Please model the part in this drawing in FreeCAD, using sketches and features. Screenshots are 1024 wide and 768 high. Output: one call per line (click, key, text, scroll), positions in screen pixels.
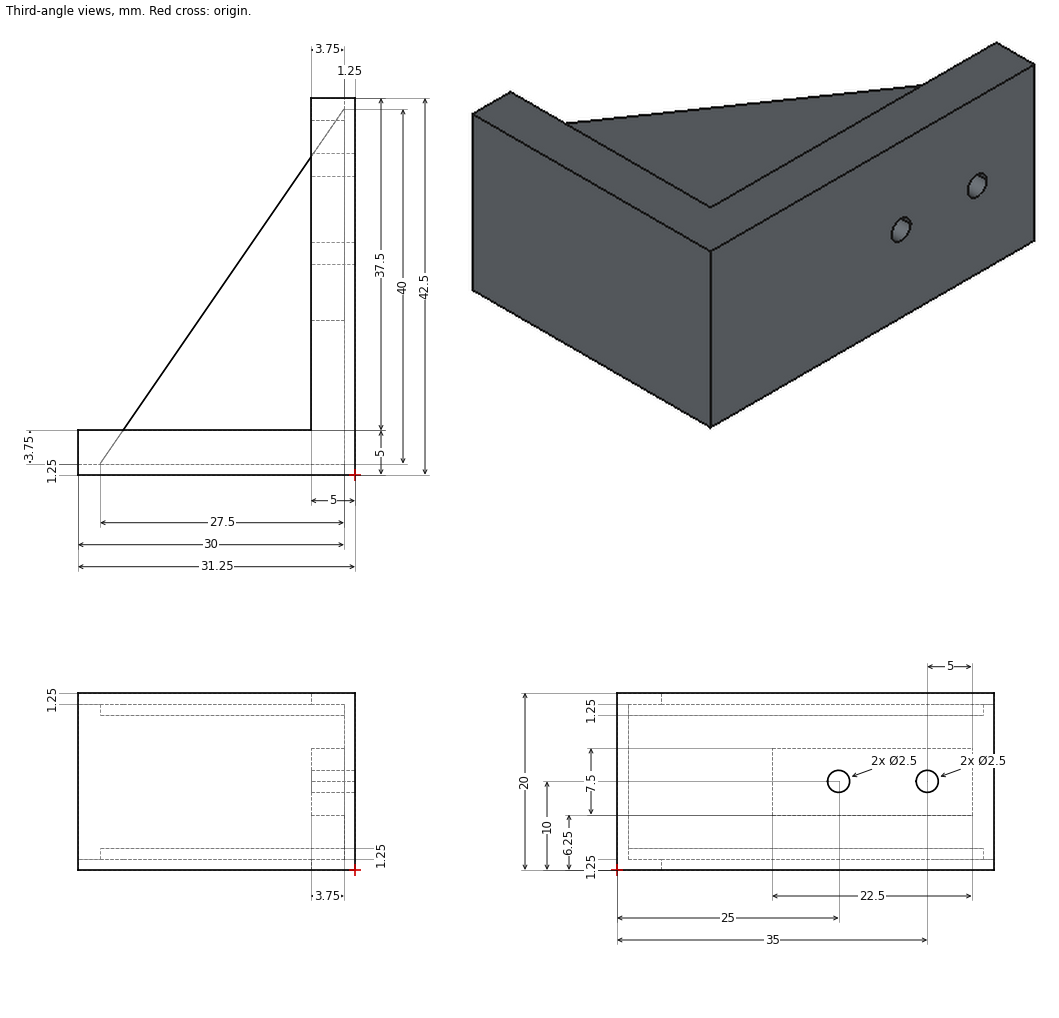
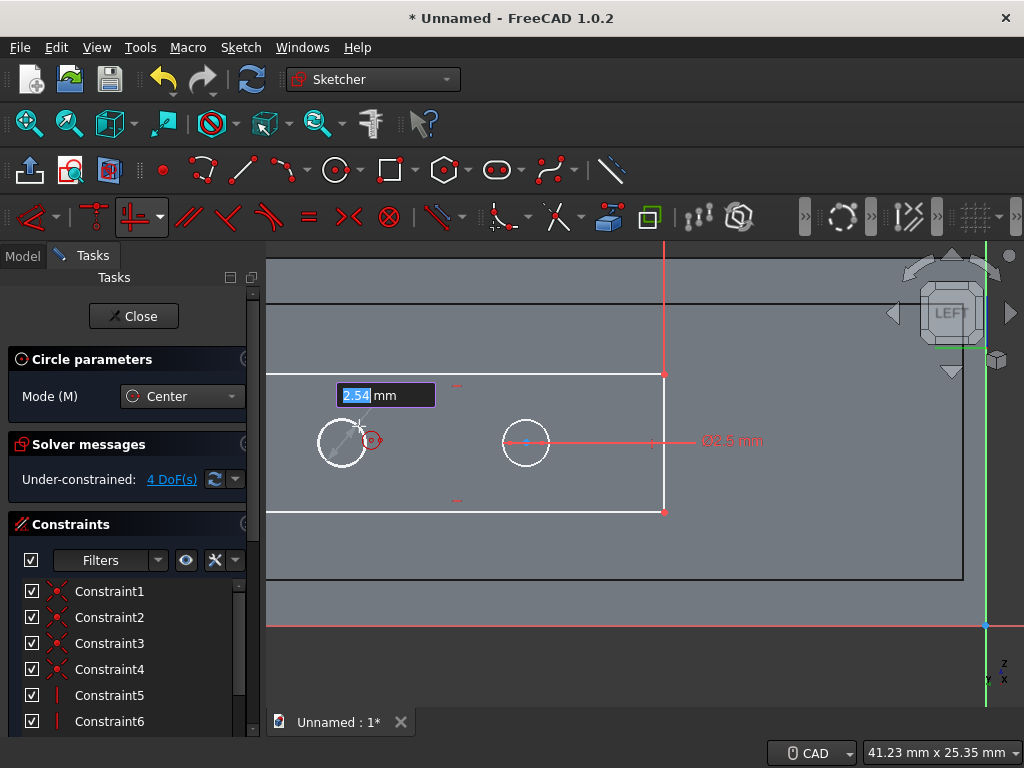
text(2.5)
key(Return)
key(Escape)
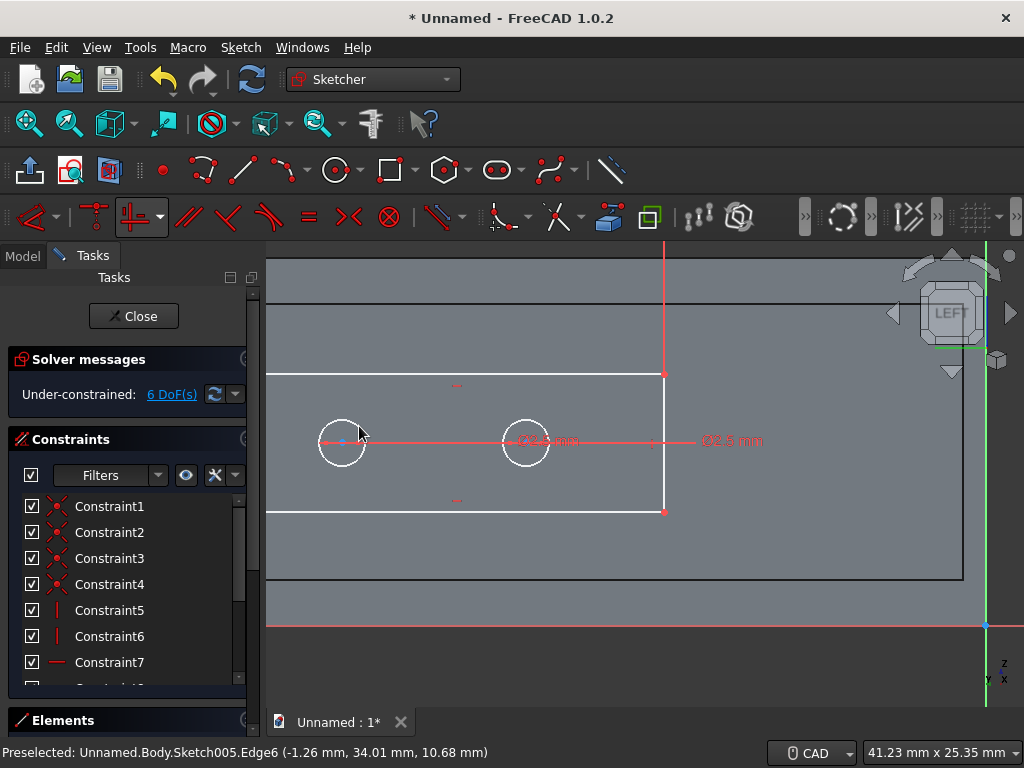
click(526, 443)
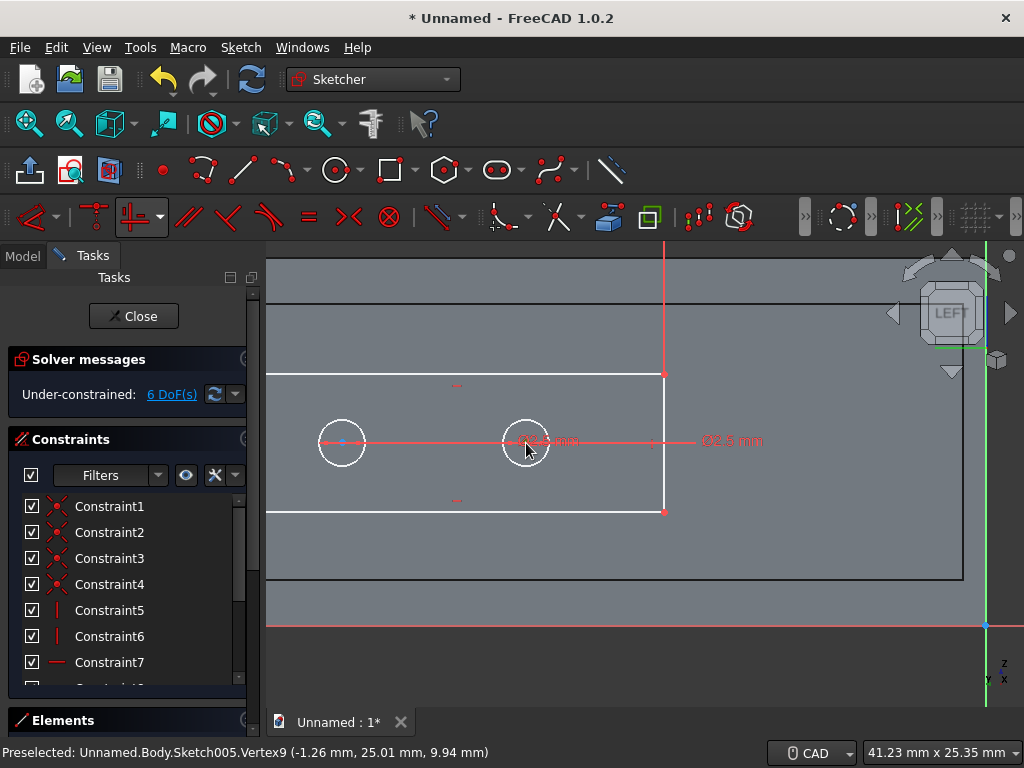
click(342, 443)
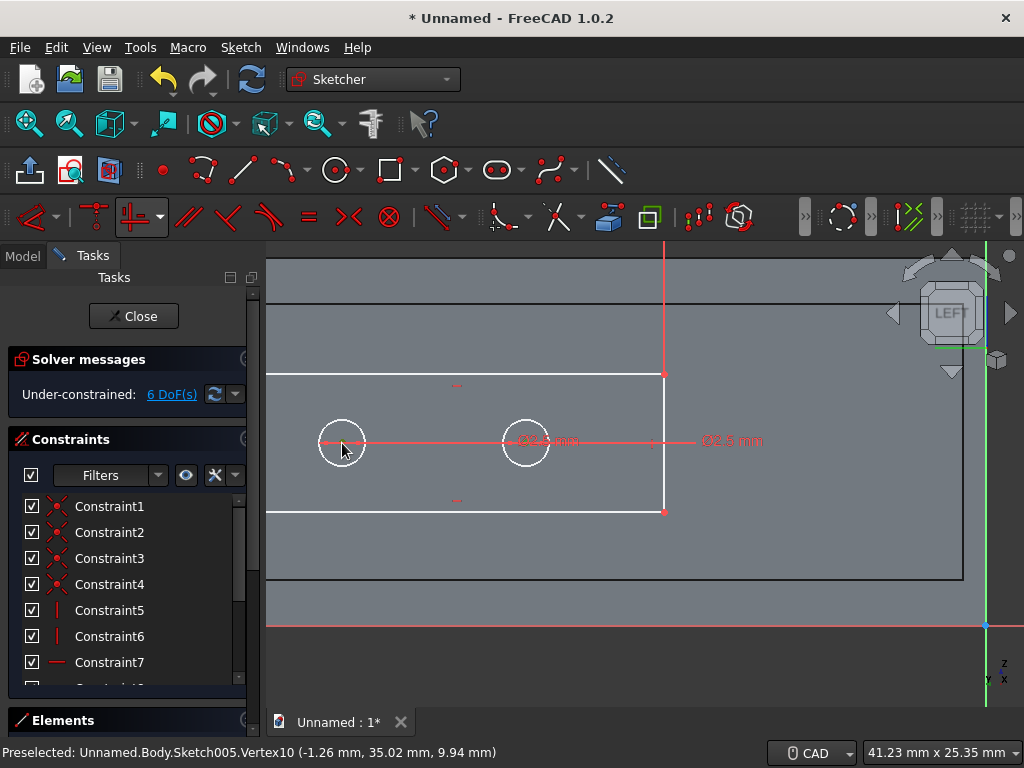
key(h)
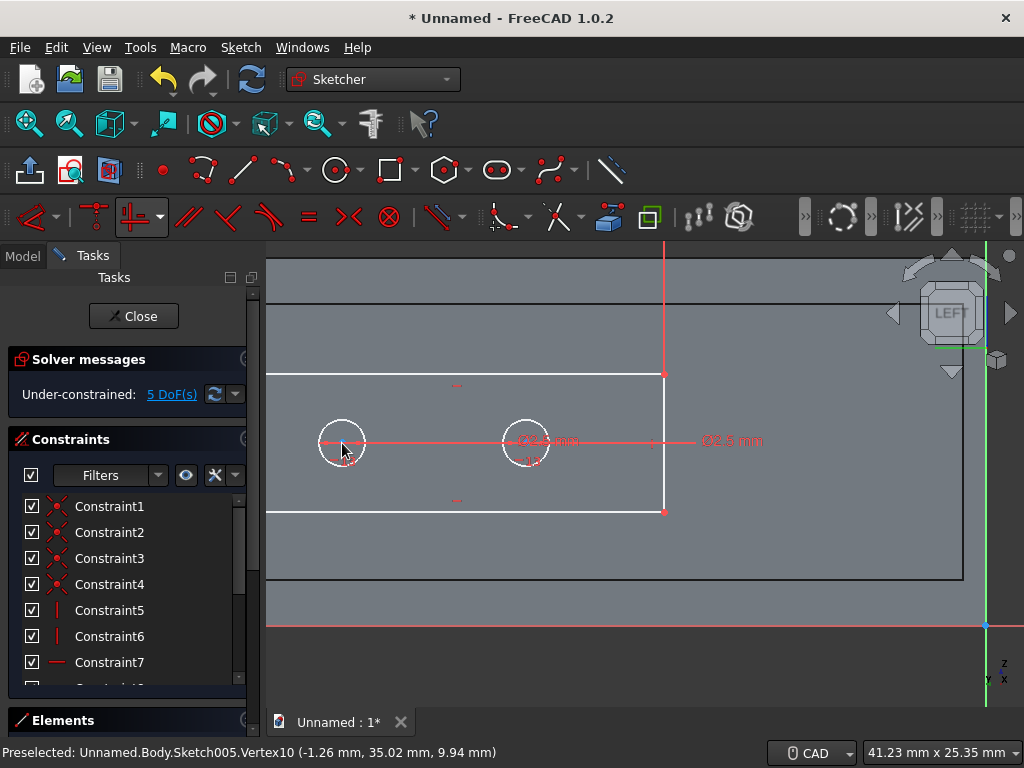
click(32, 218)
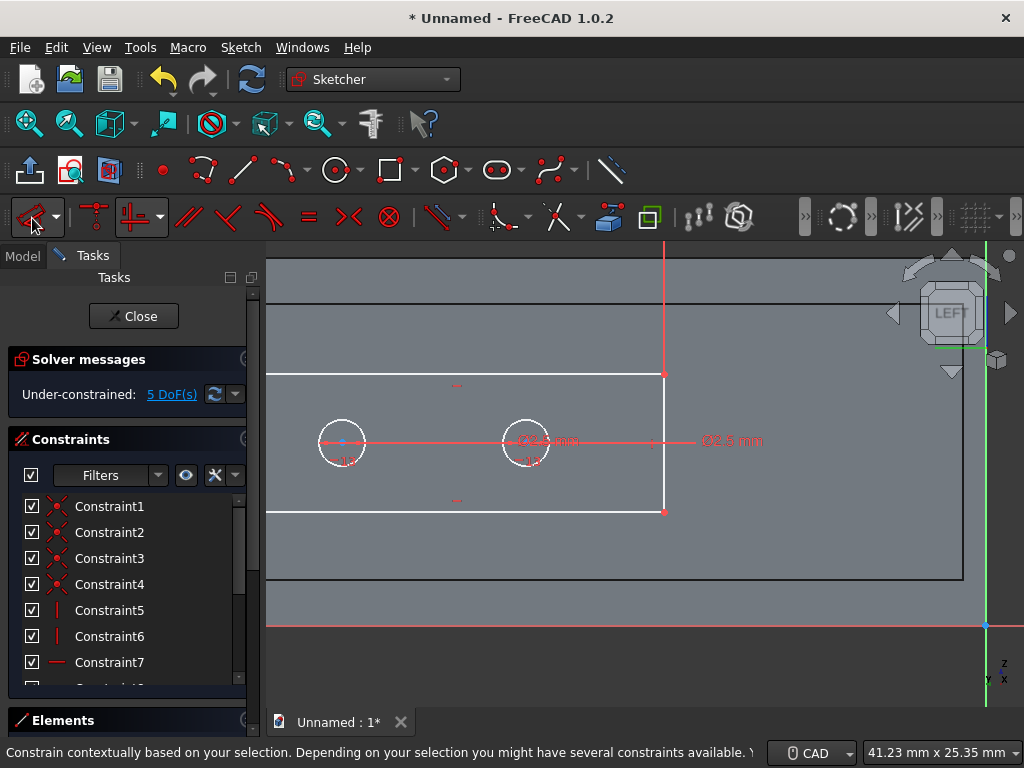
click(526, 443)
click(692, 660)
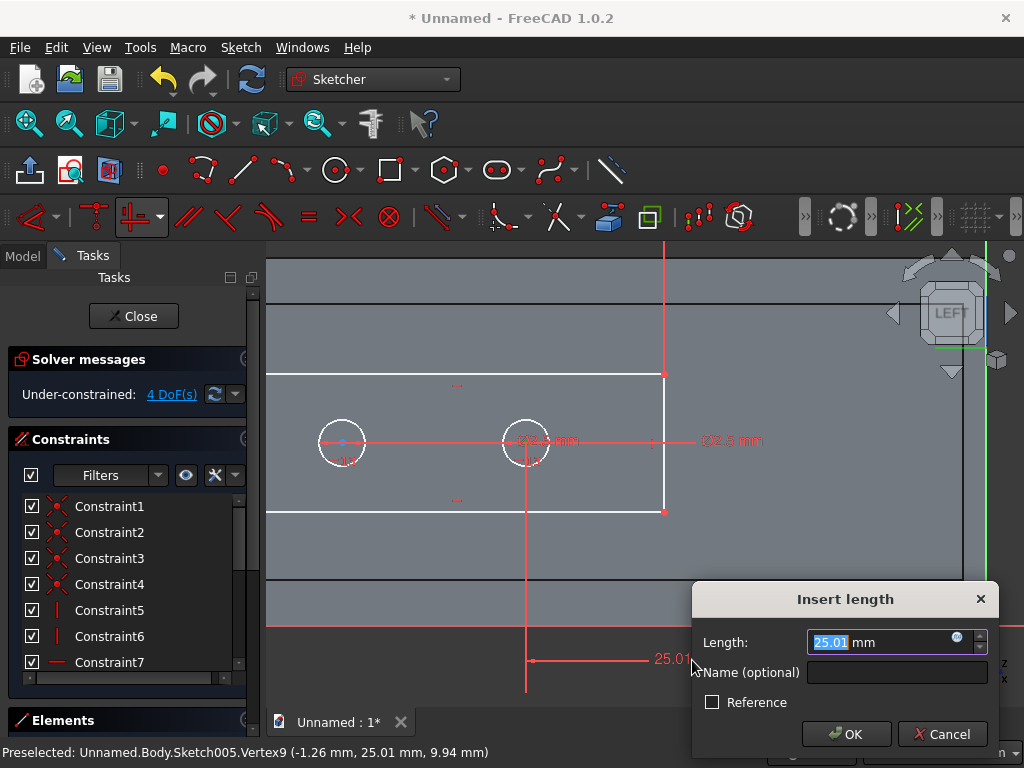
text(25)
key(Return)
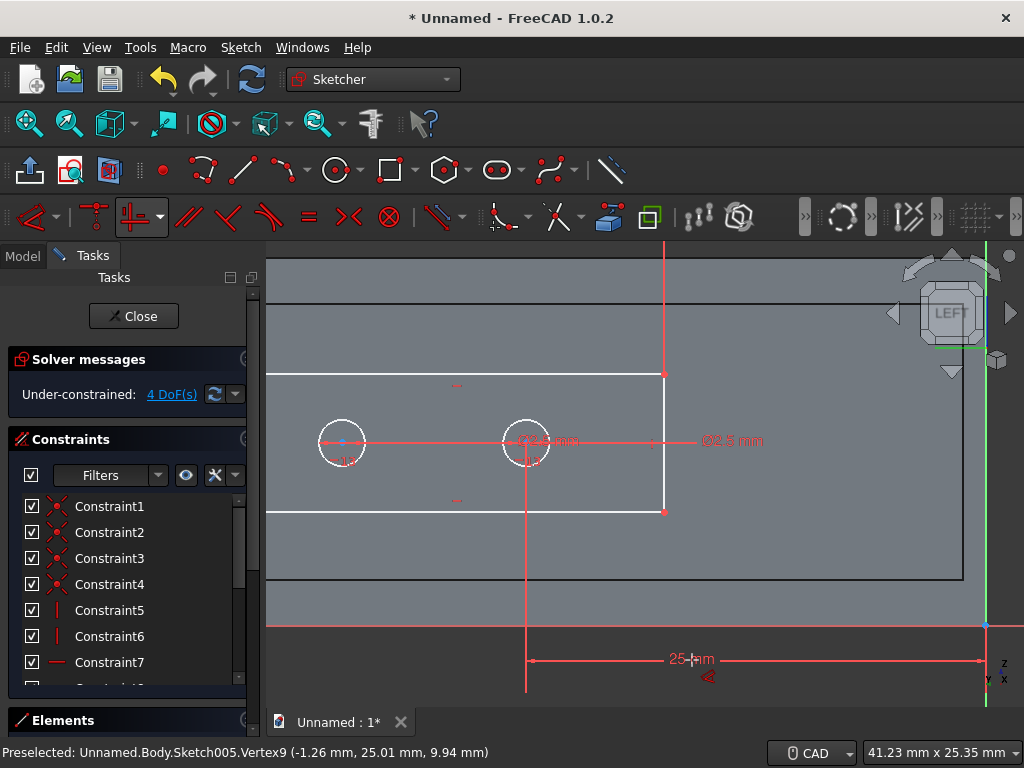
click(526, 443)
click(492, 534)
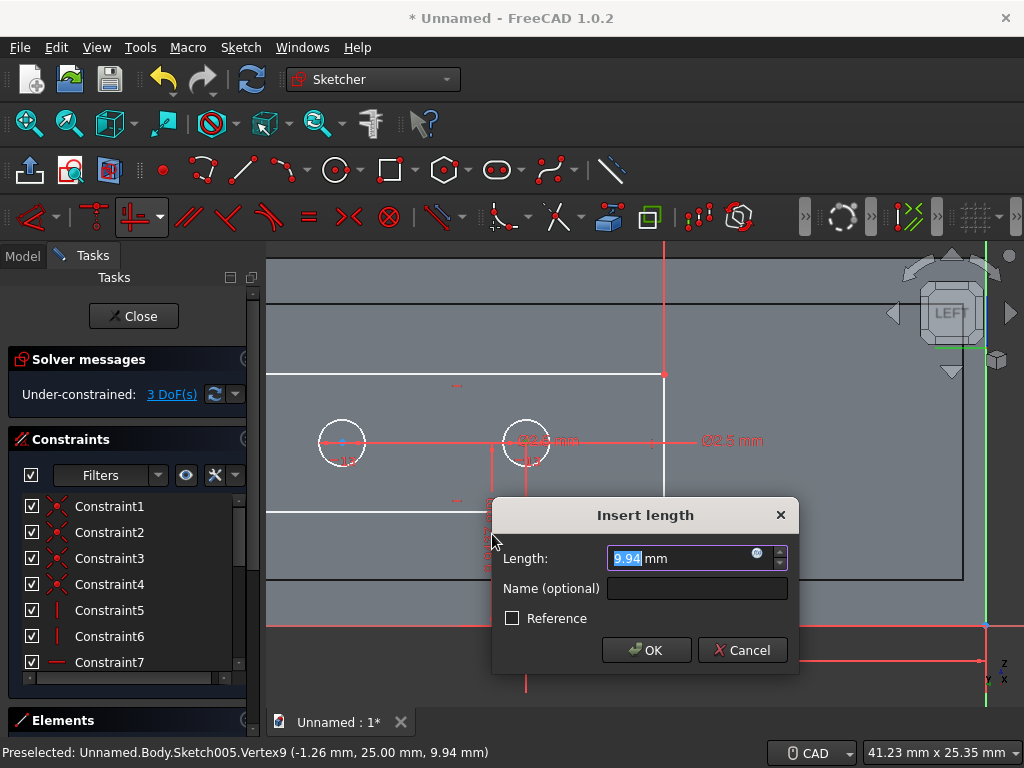
text(10)
key(Return)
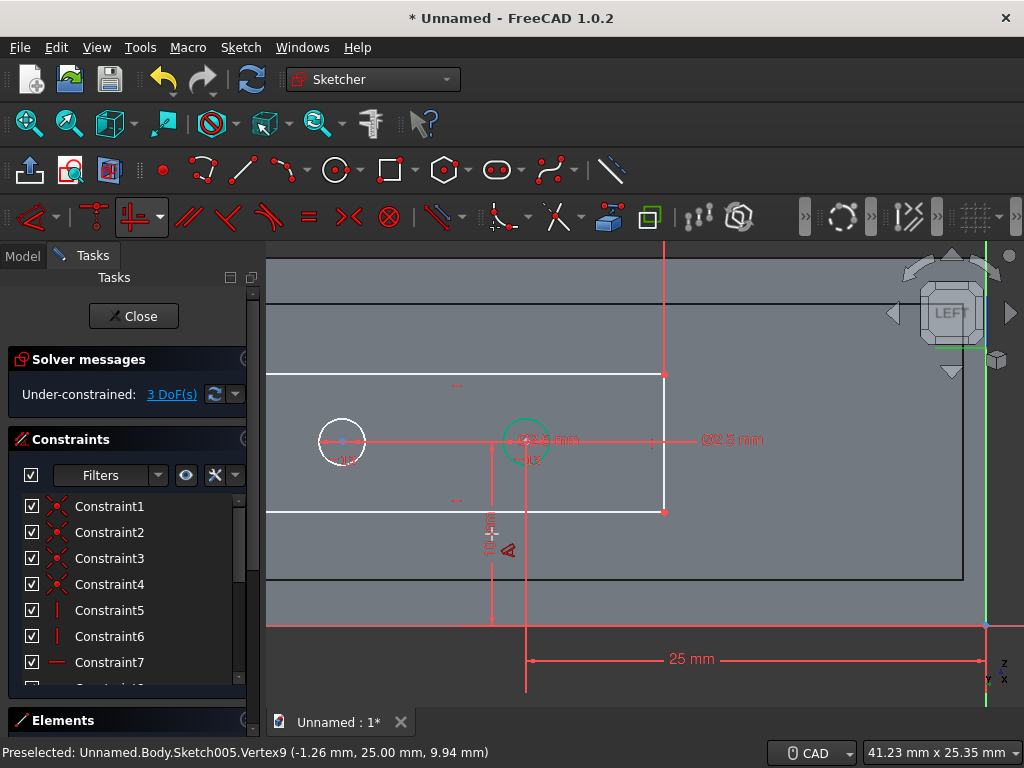
click(342, 442)
click(600, 660)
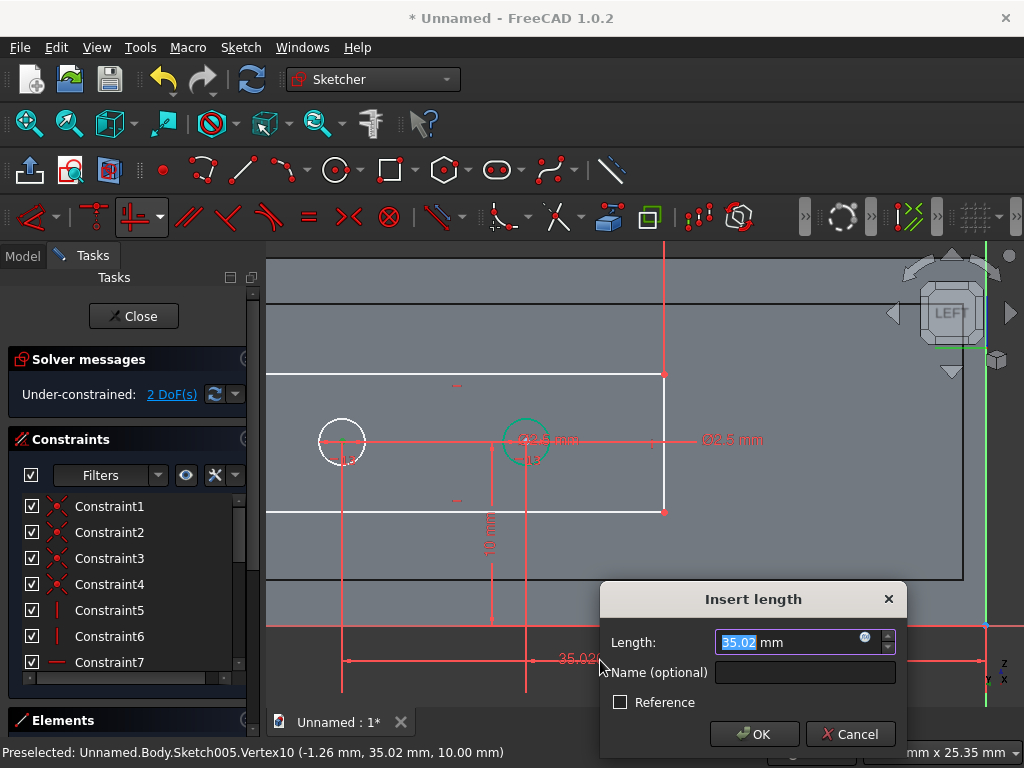
text(35)
key(Return)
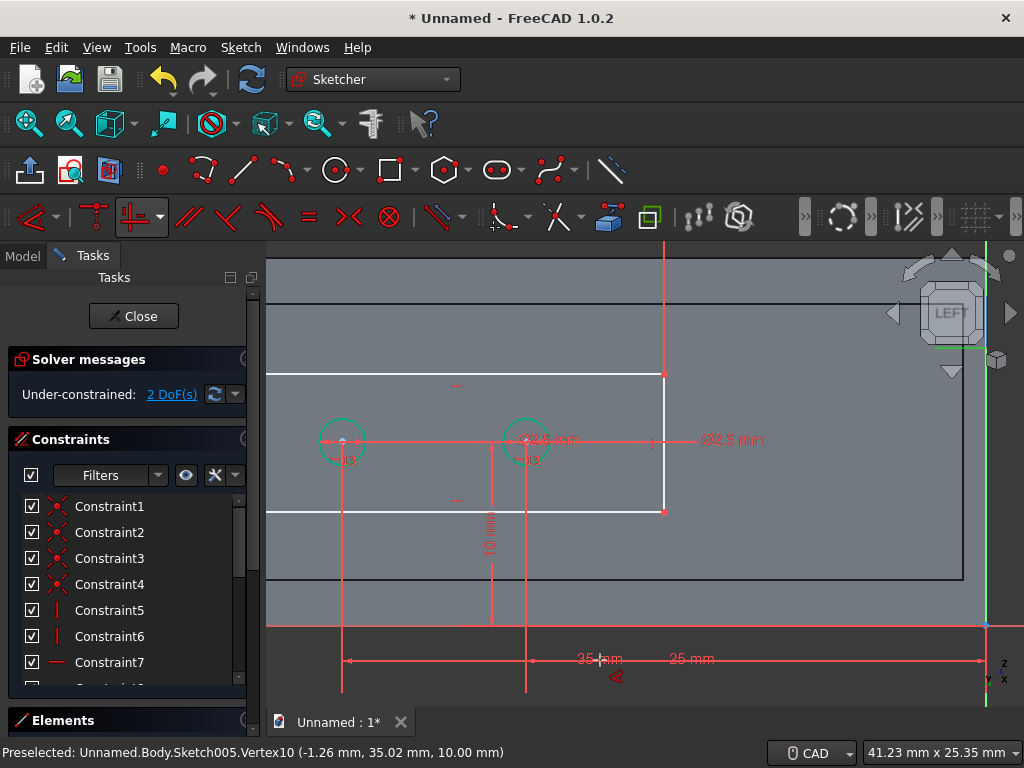
scroll(526, 443, down, 3)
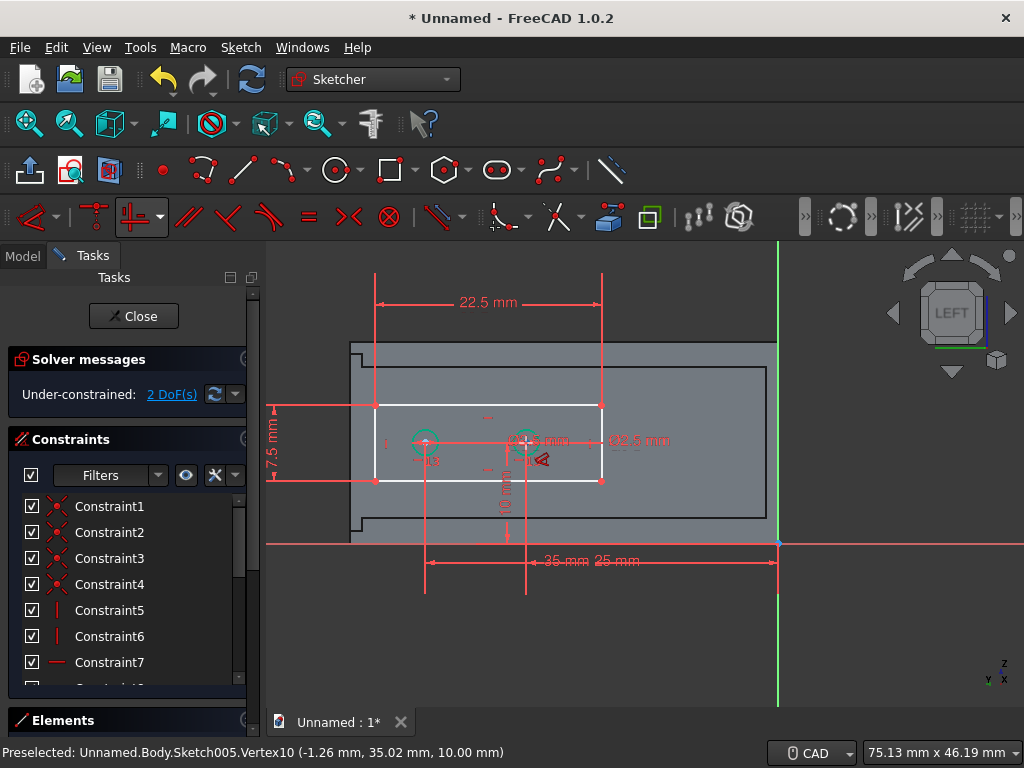
click(375, 405)